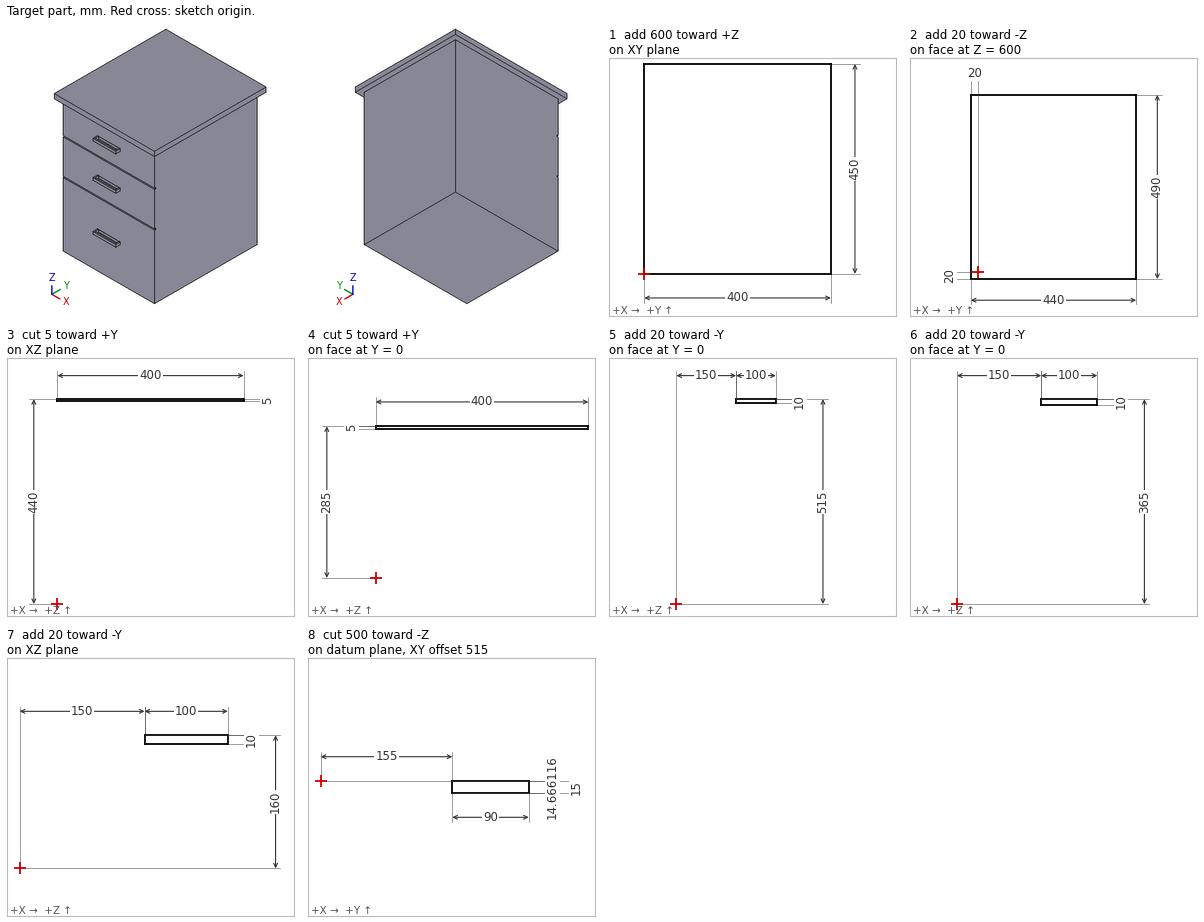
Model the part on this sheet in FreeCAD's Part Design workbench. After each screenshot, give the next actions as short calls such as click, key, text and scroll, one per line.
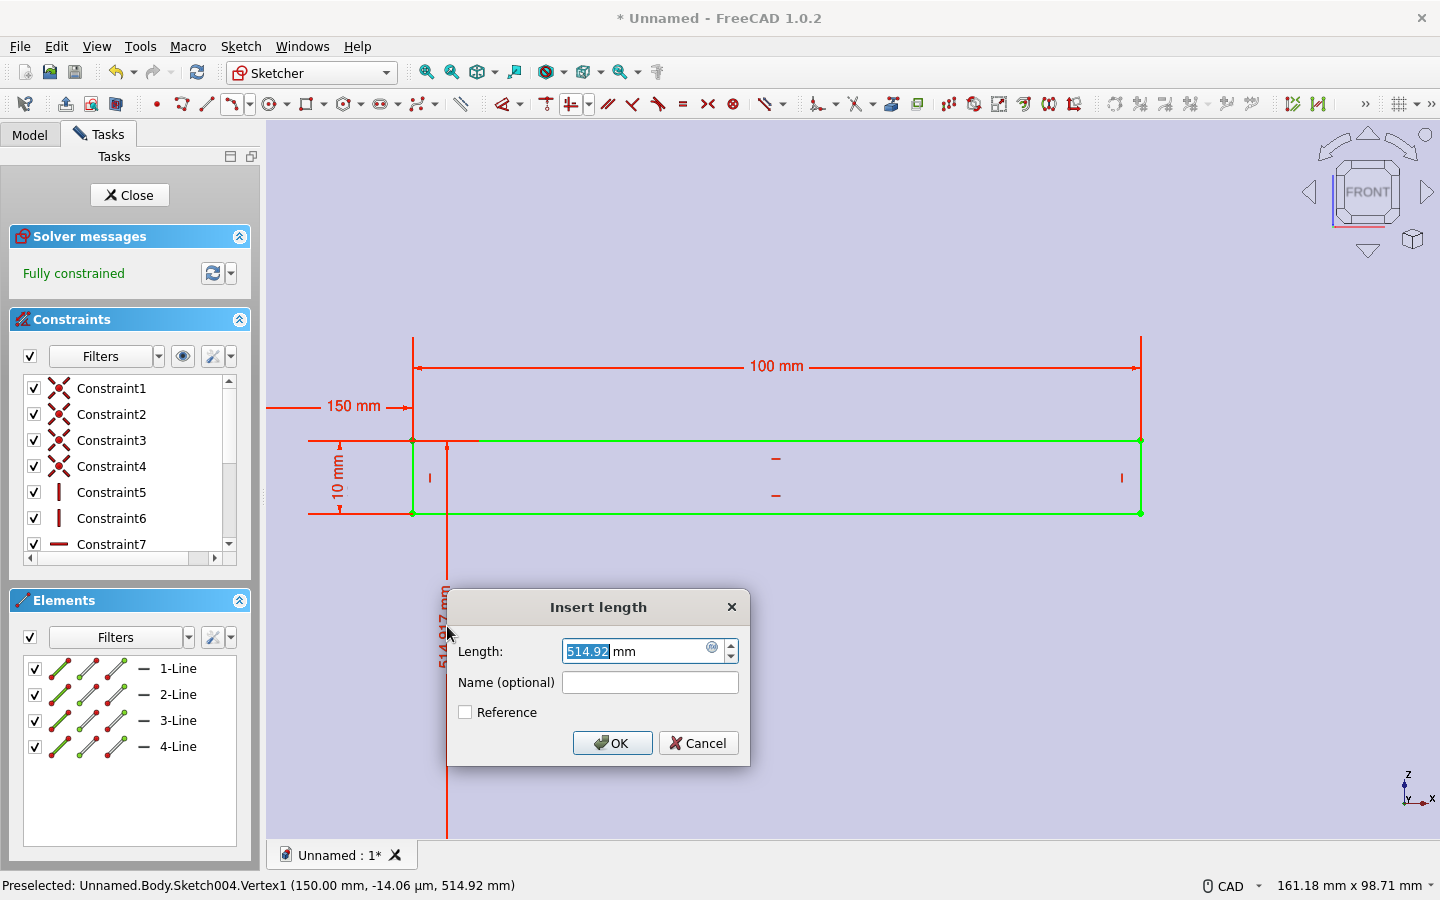
text(515)
key(Return)
key(Escape)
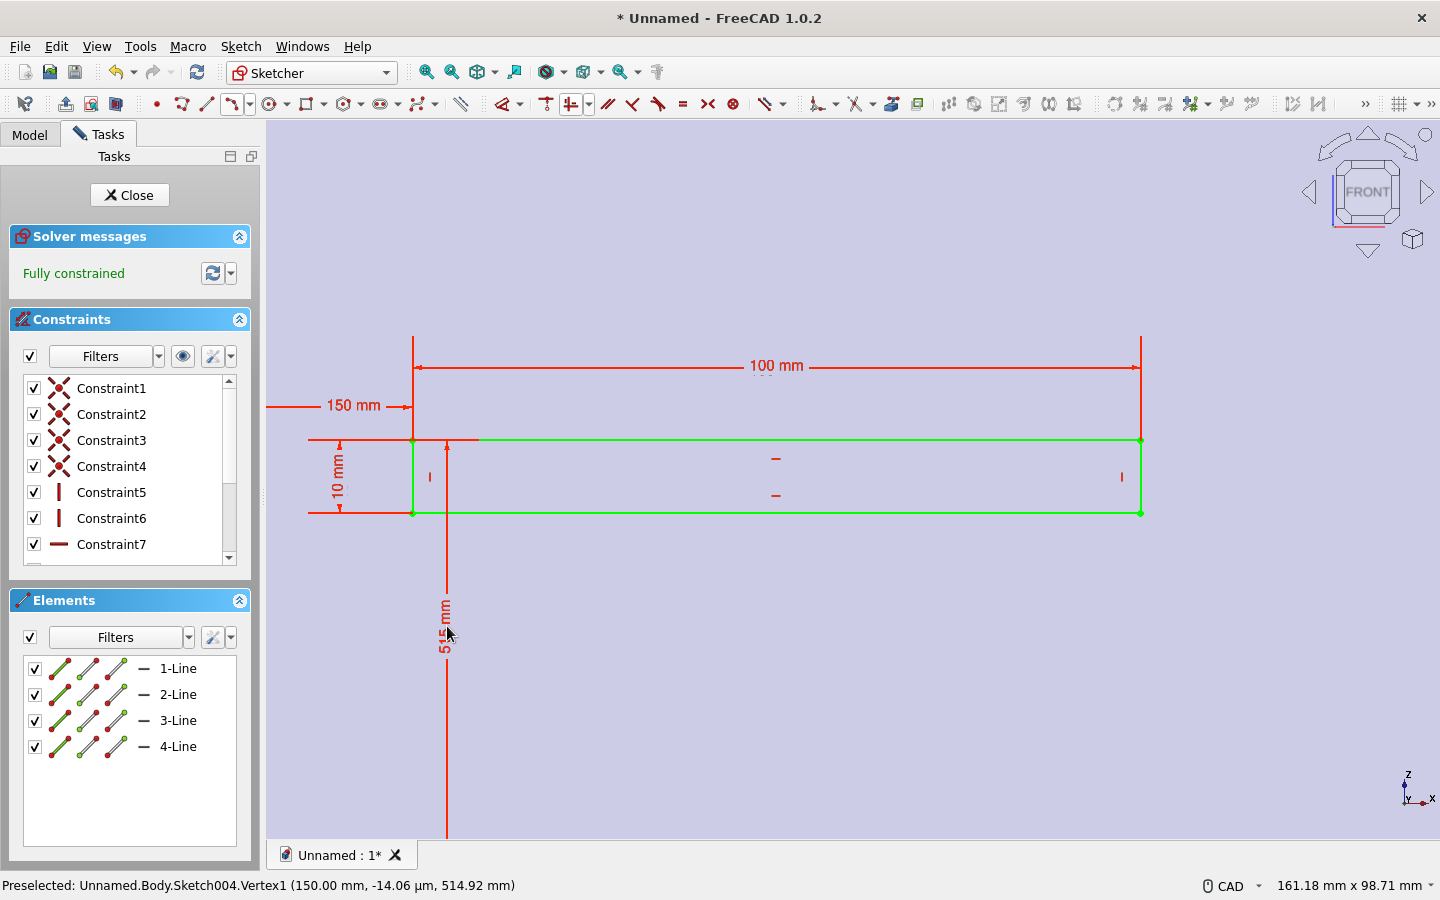
click(130, 195)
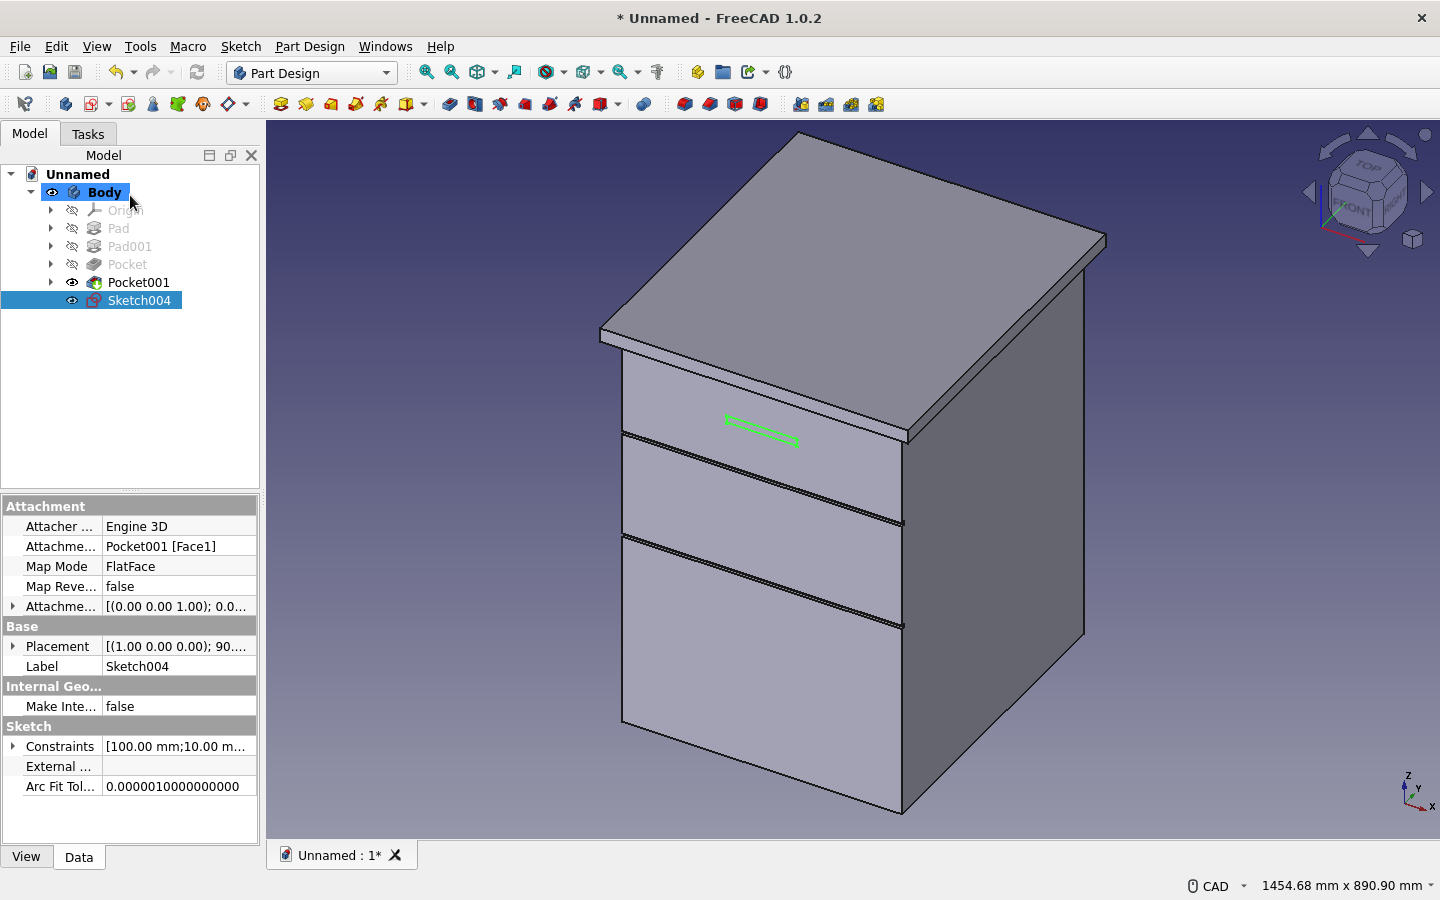
click(281, 104)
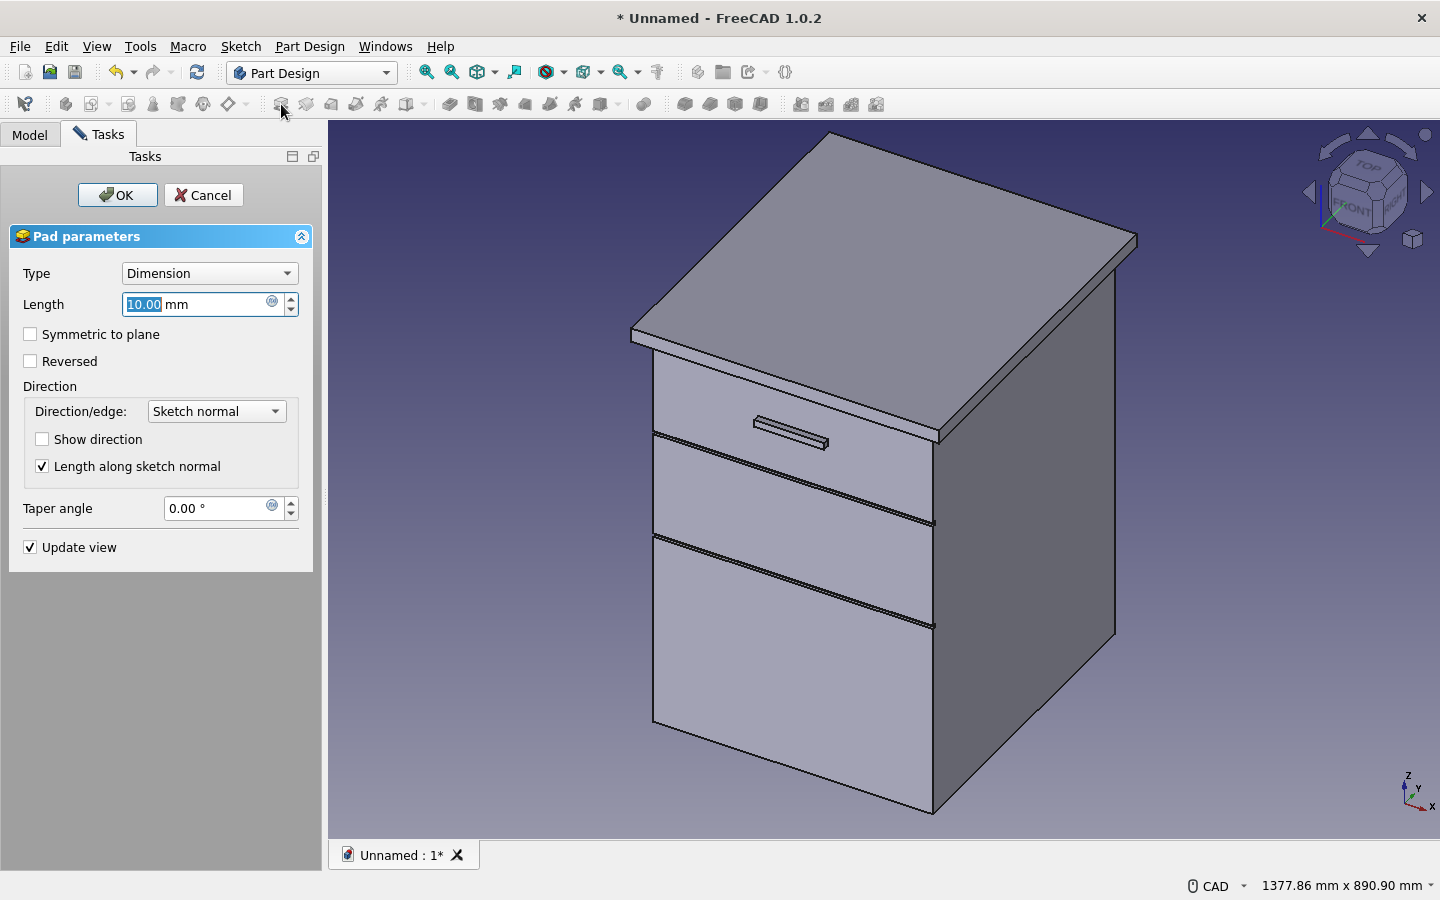
text(20)
key(Tab)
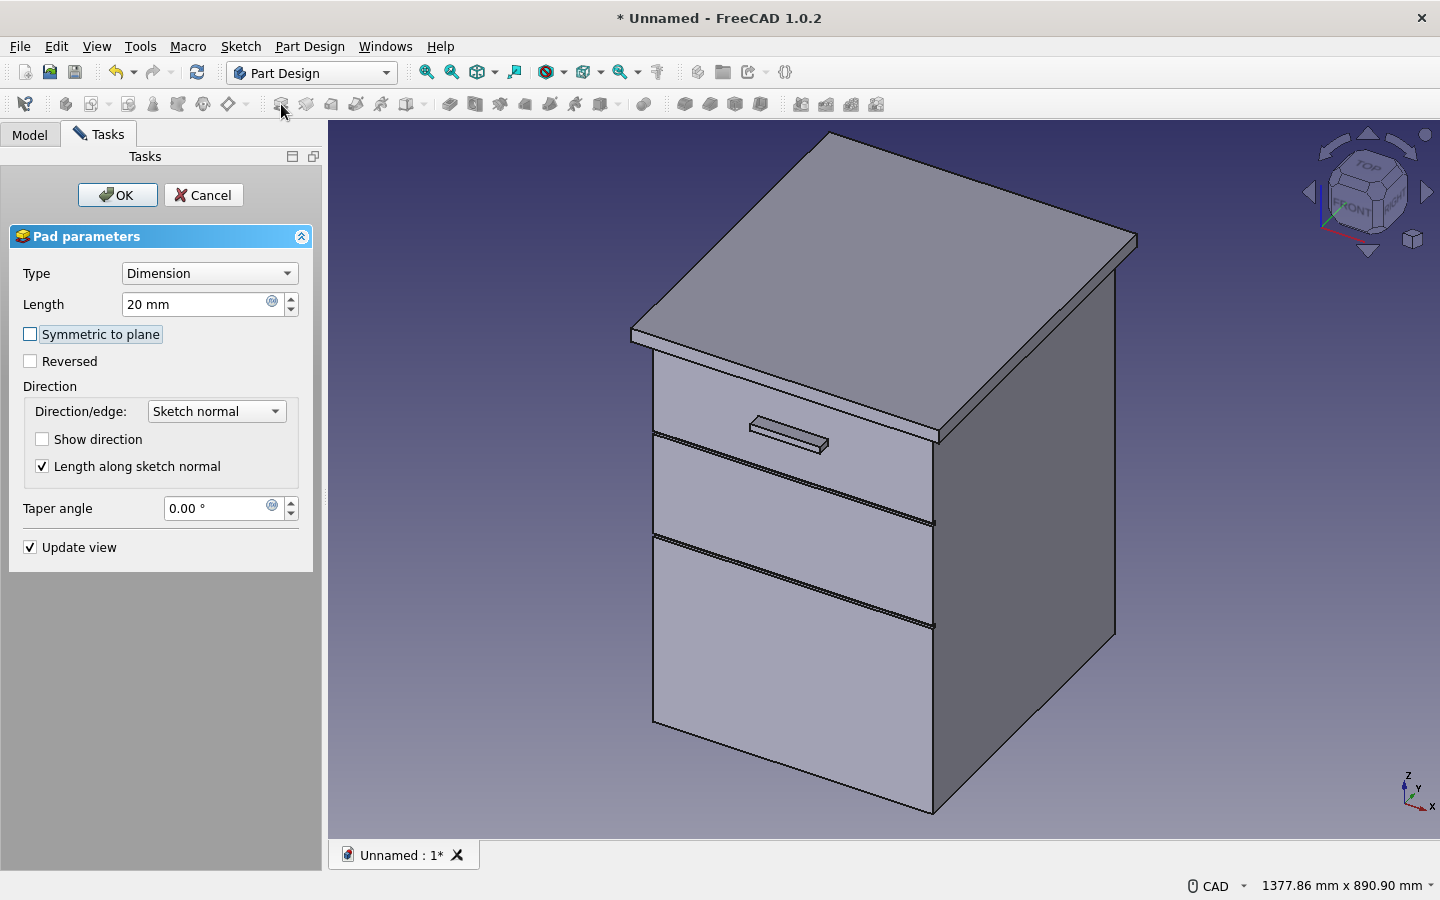
click(118, 195)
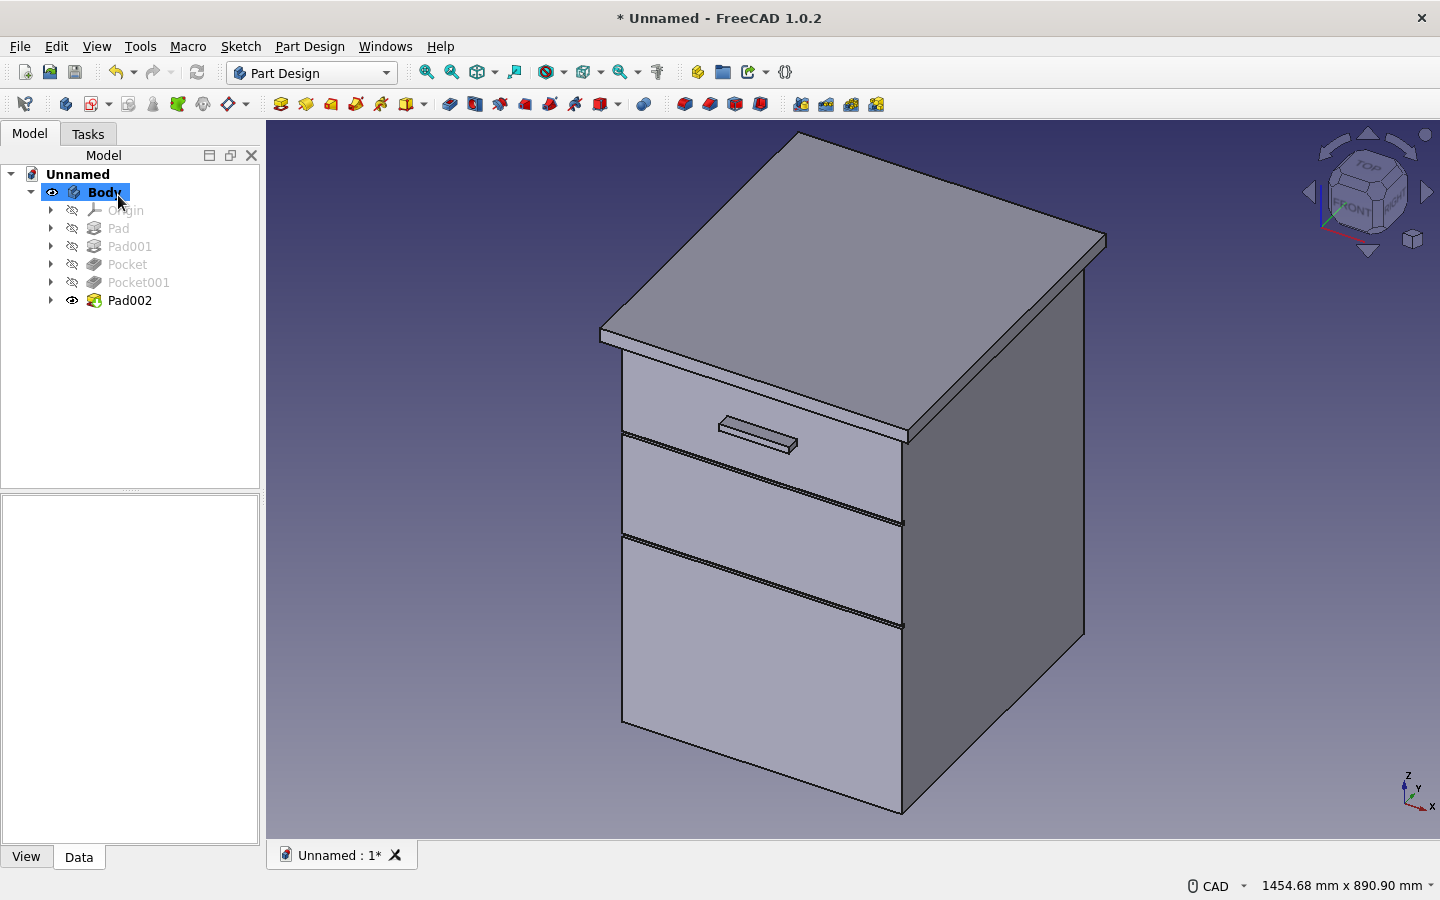
click(802, 688)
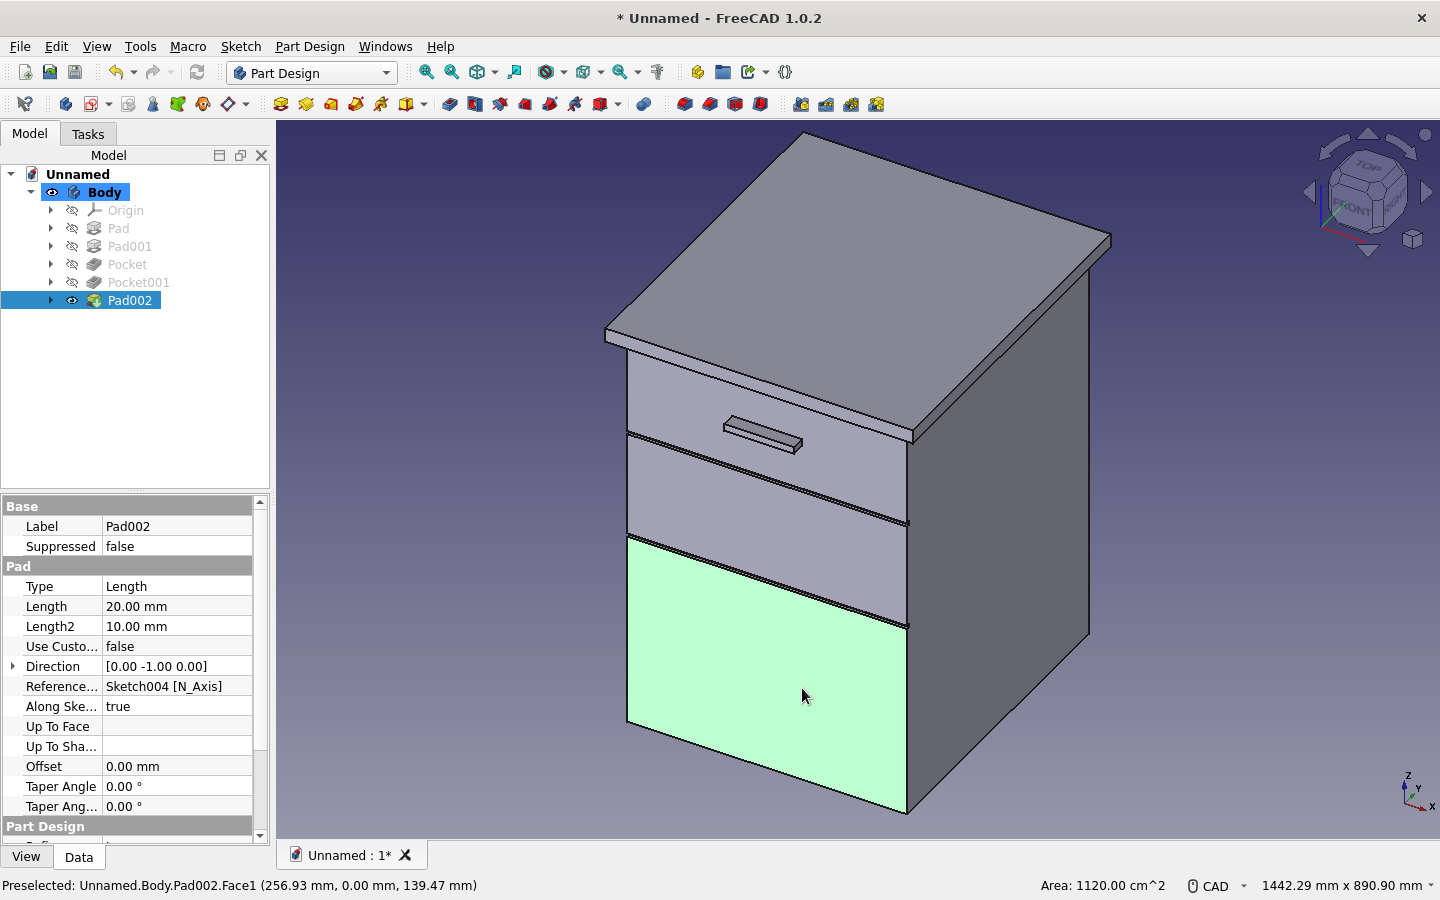
click(90, 104)